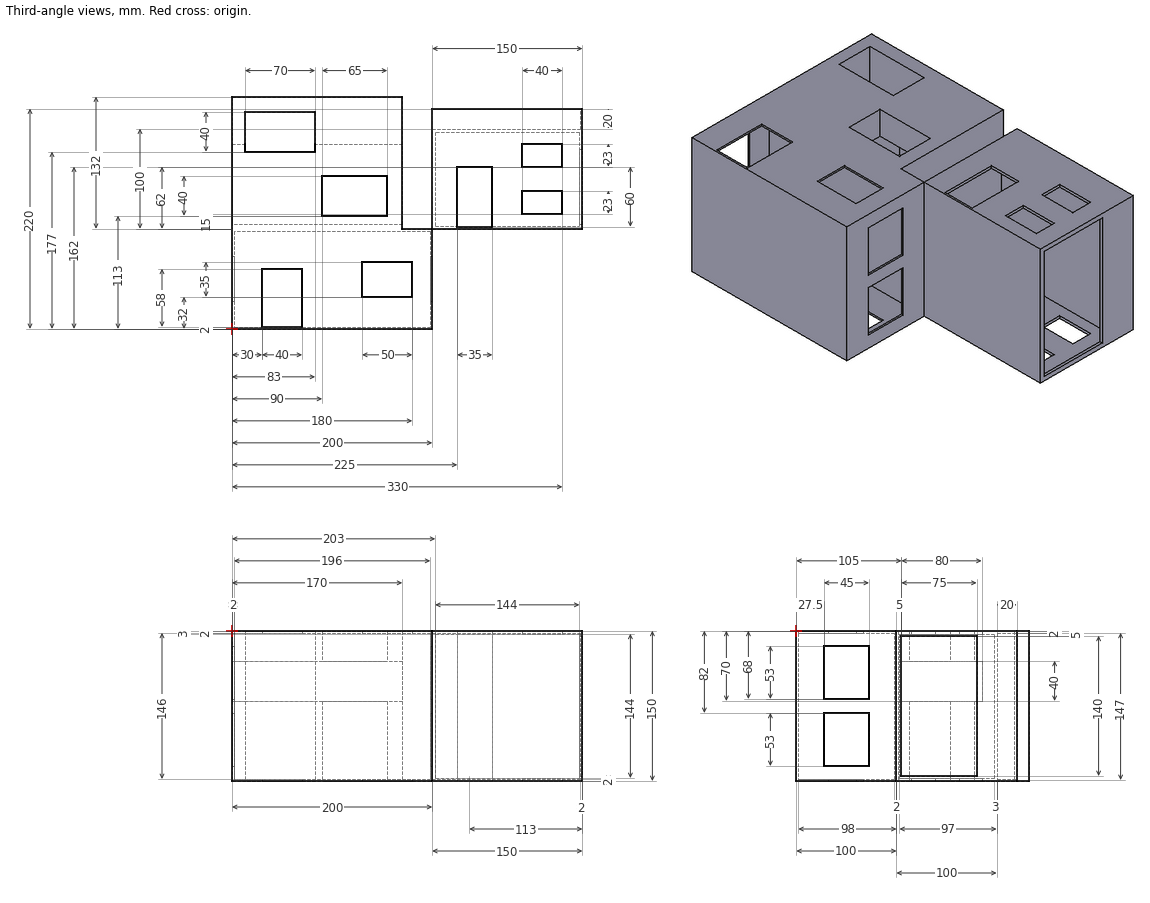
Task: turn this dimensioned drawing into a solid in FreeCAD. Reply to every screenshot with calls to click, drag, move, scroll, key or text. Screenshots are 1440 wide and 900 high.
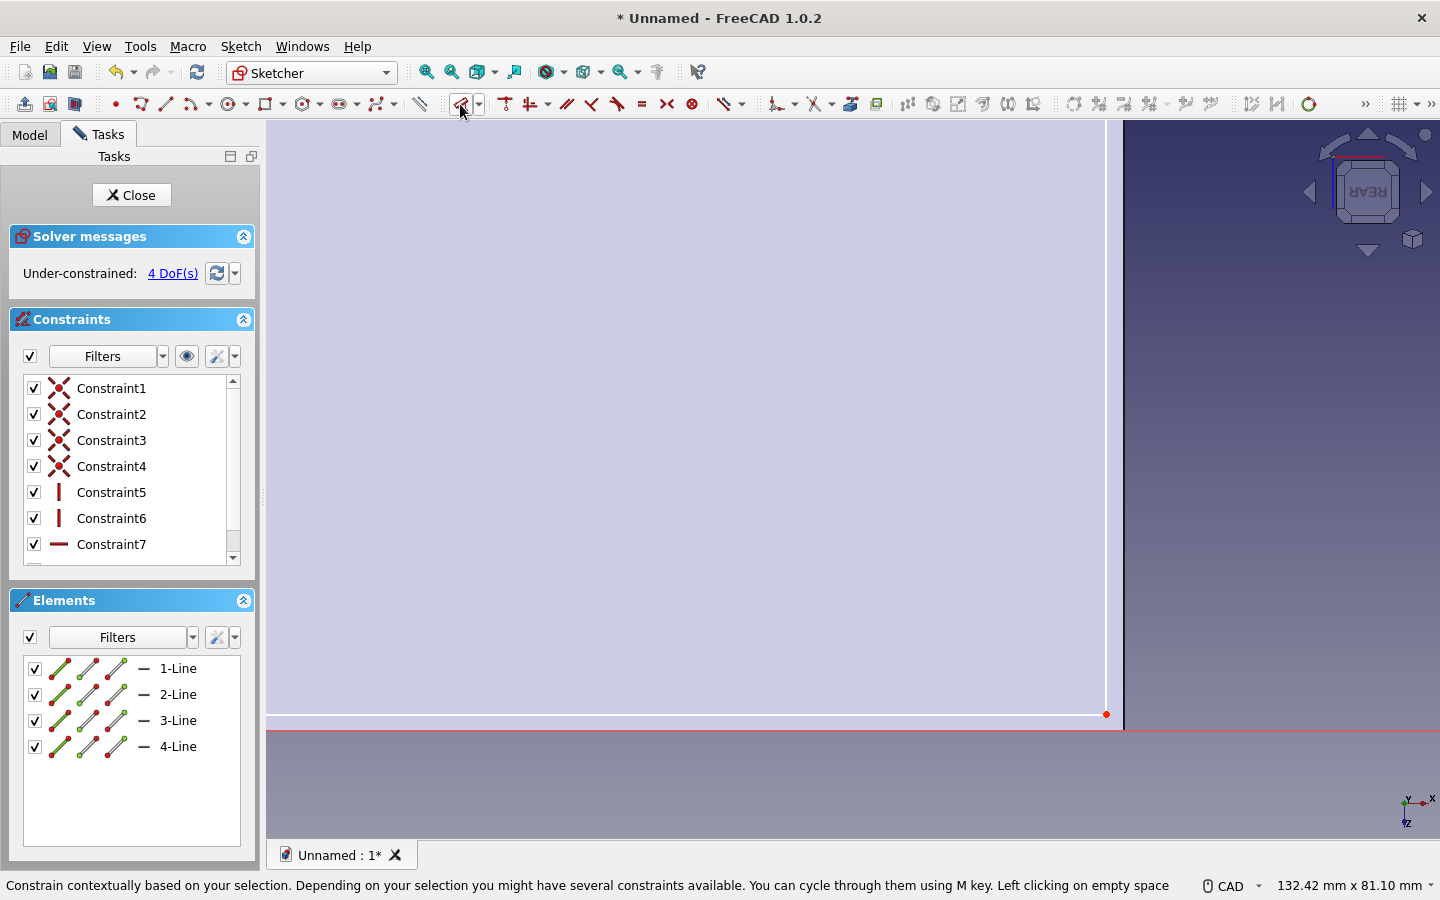
scroll(1108, 715, down, 5)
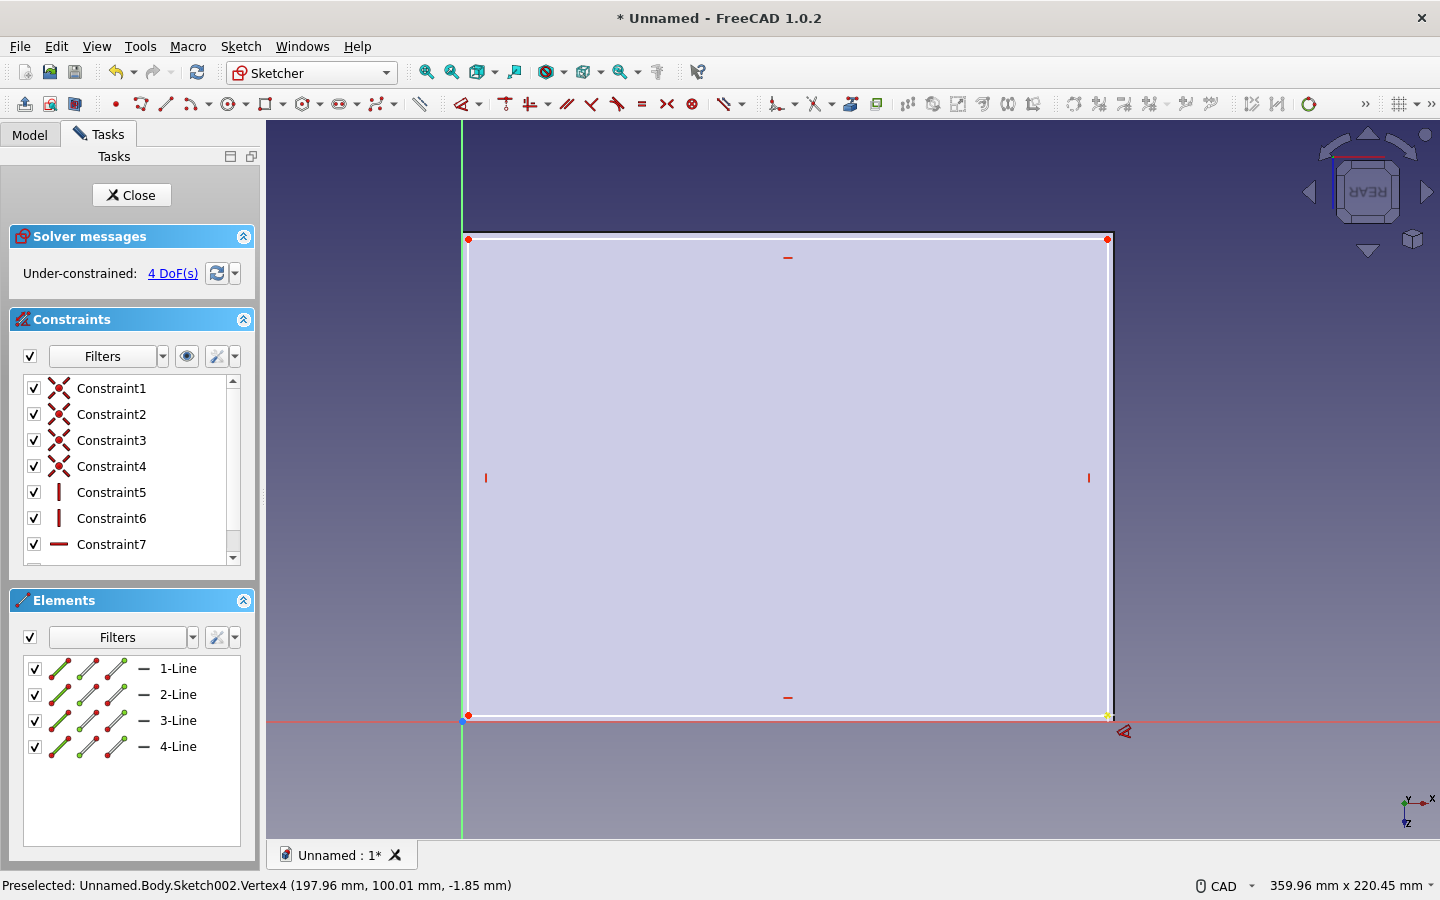
scroll(468, 239, up, 10)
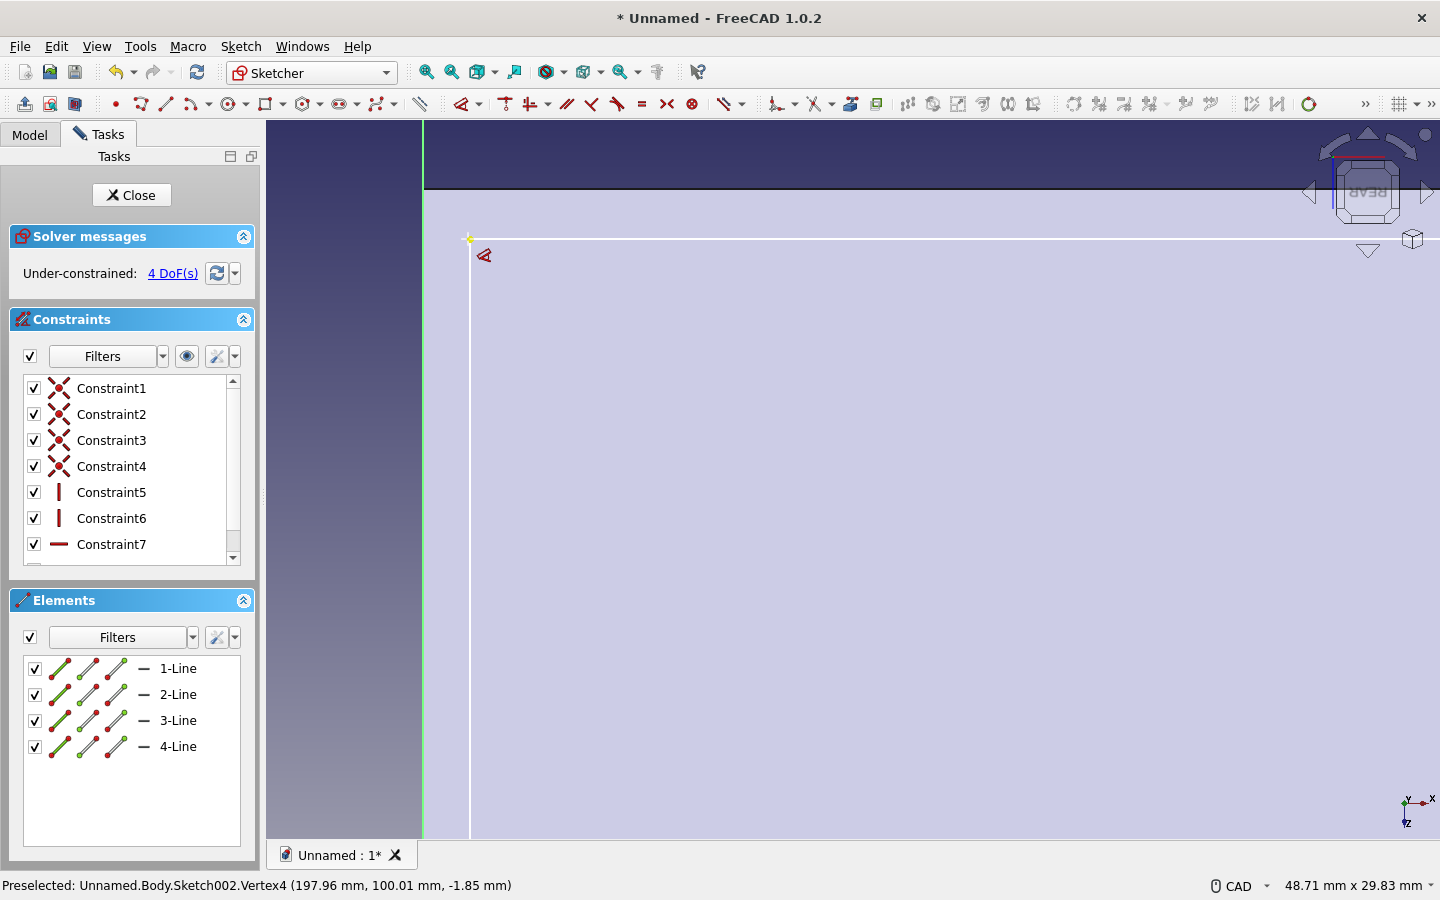
click(470, 239)
click(447, 205)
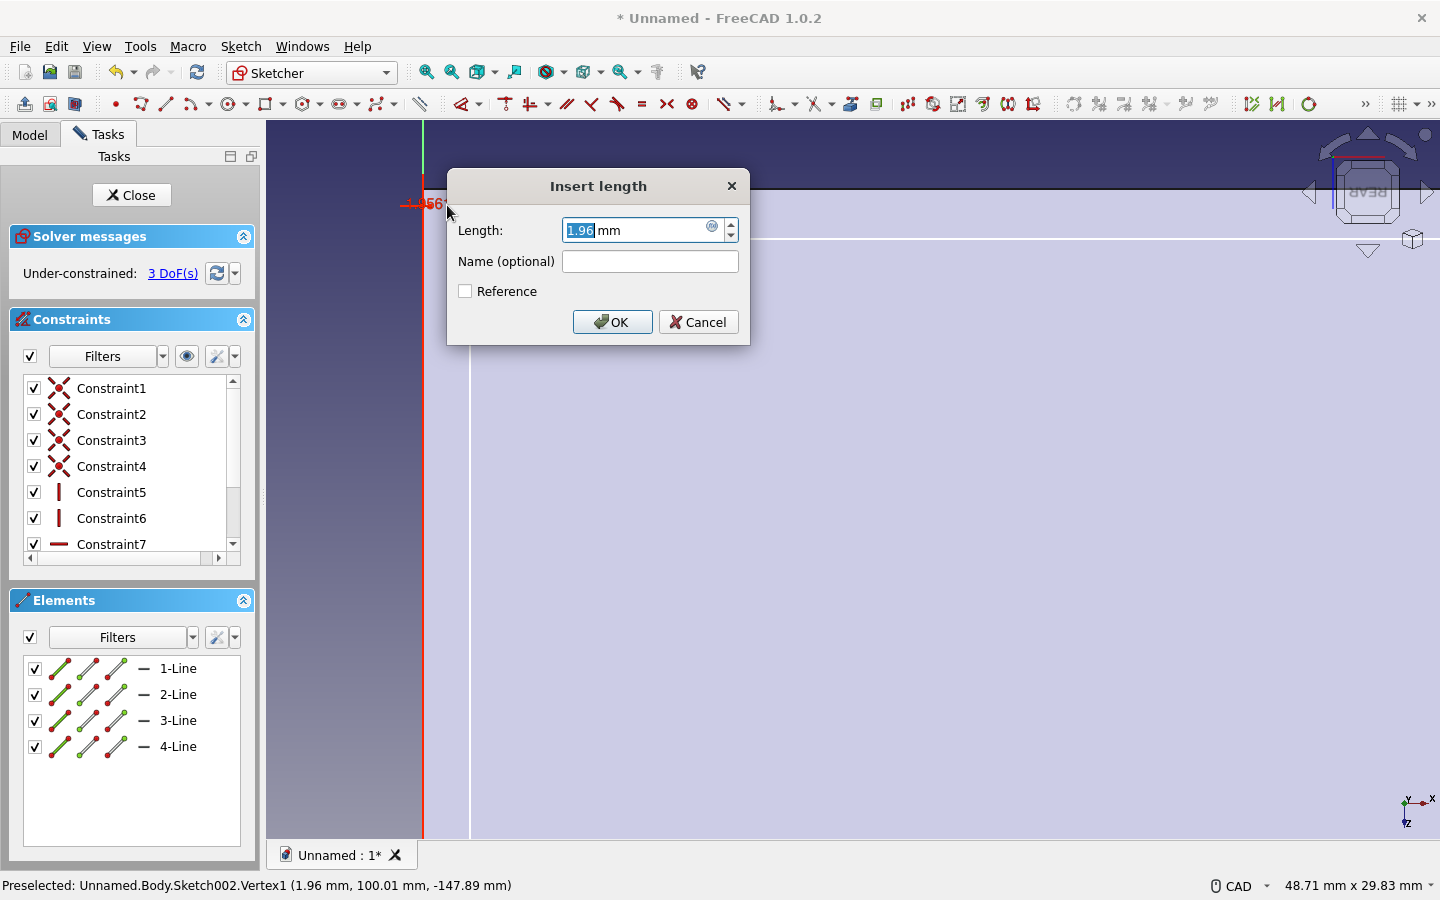
text(2)
key(Return)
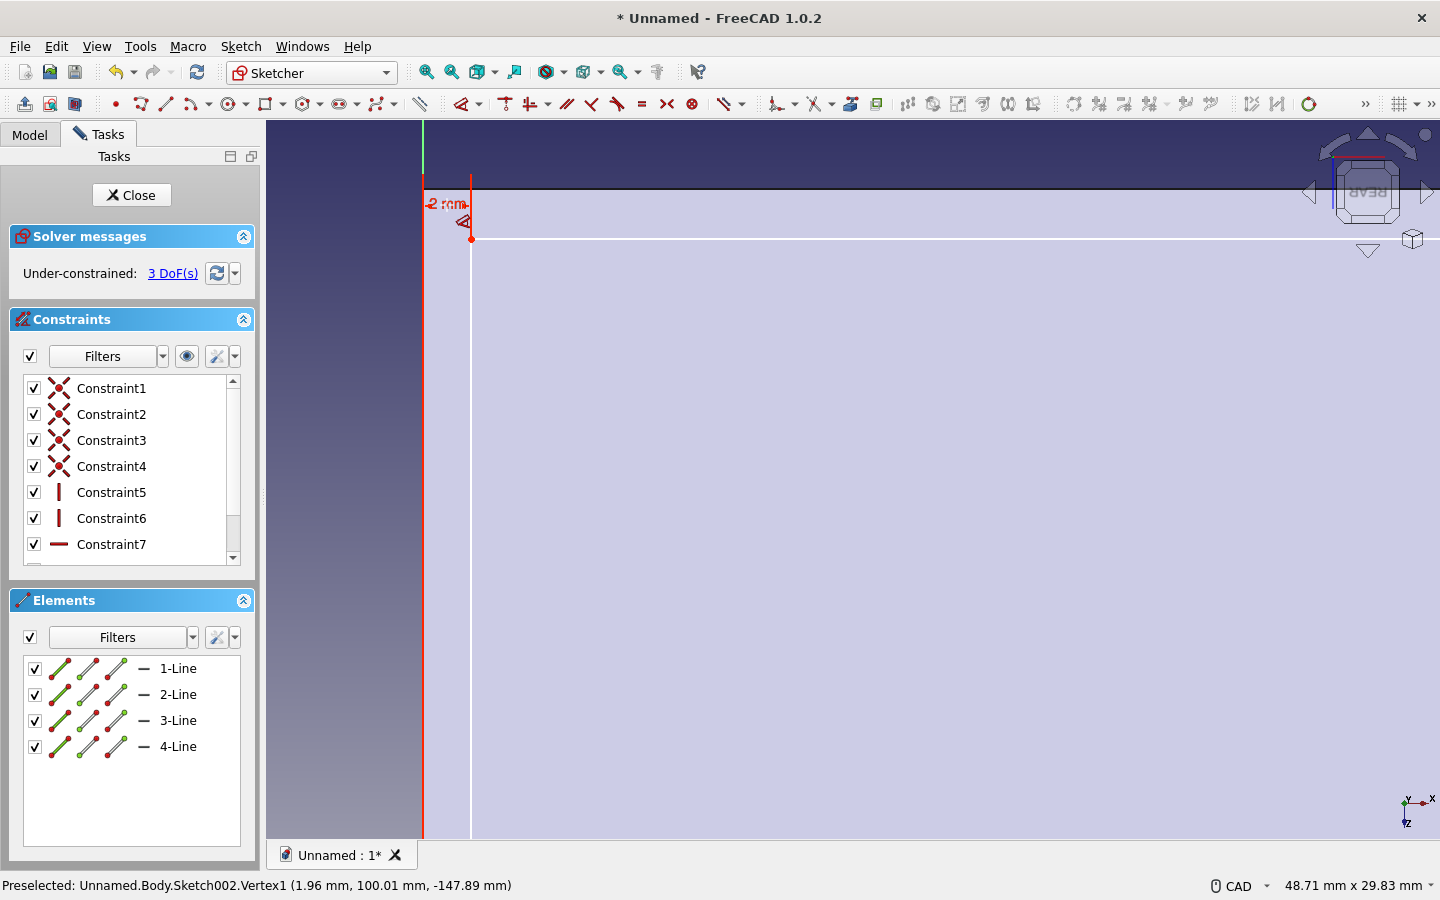
scroll(468, 238, down, 10)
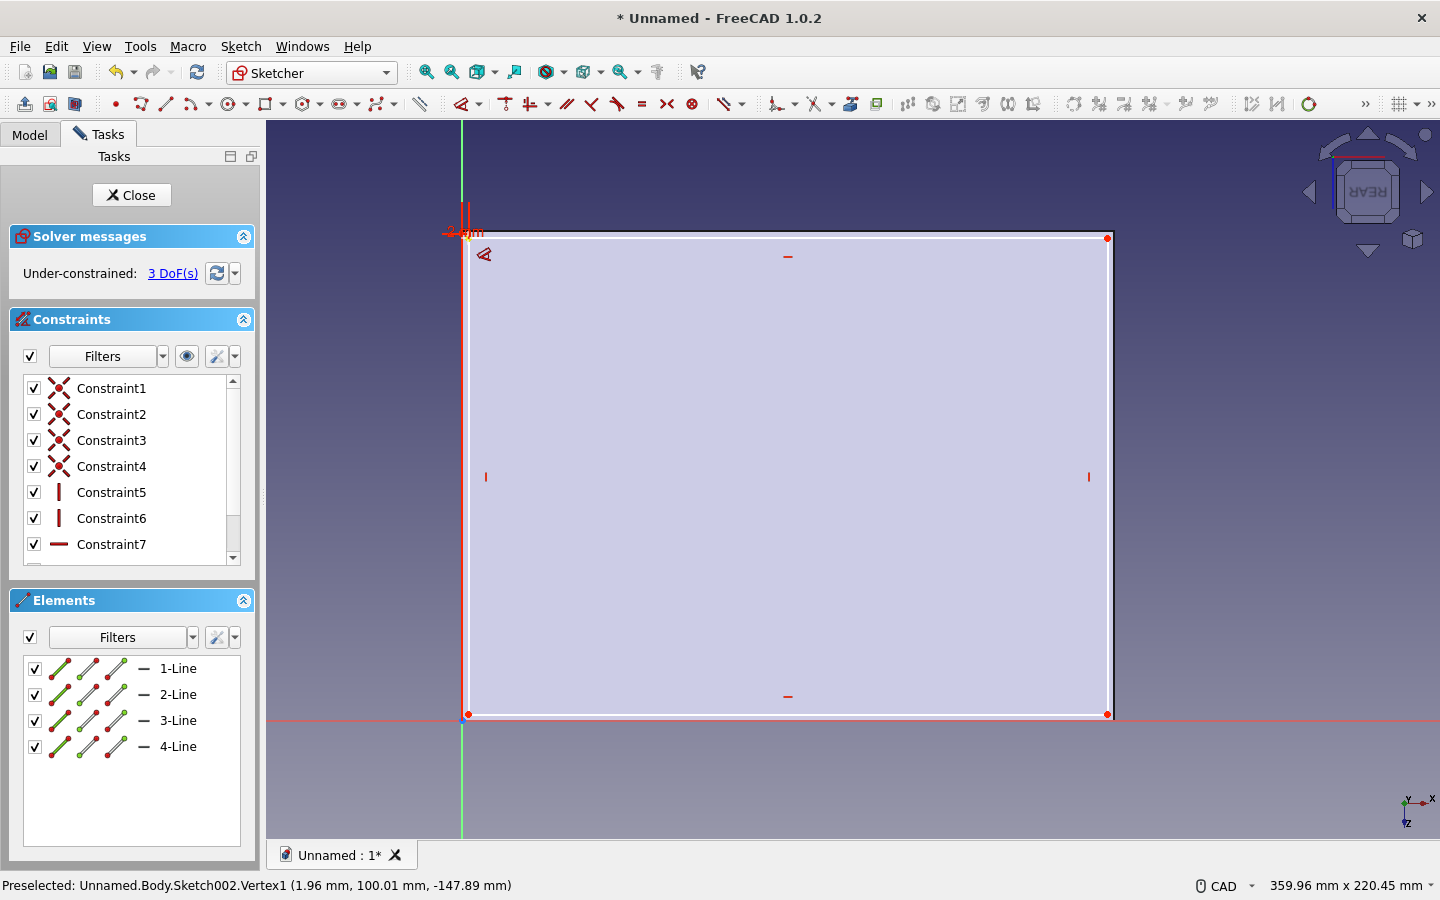
scroll(469, 715, up, 10)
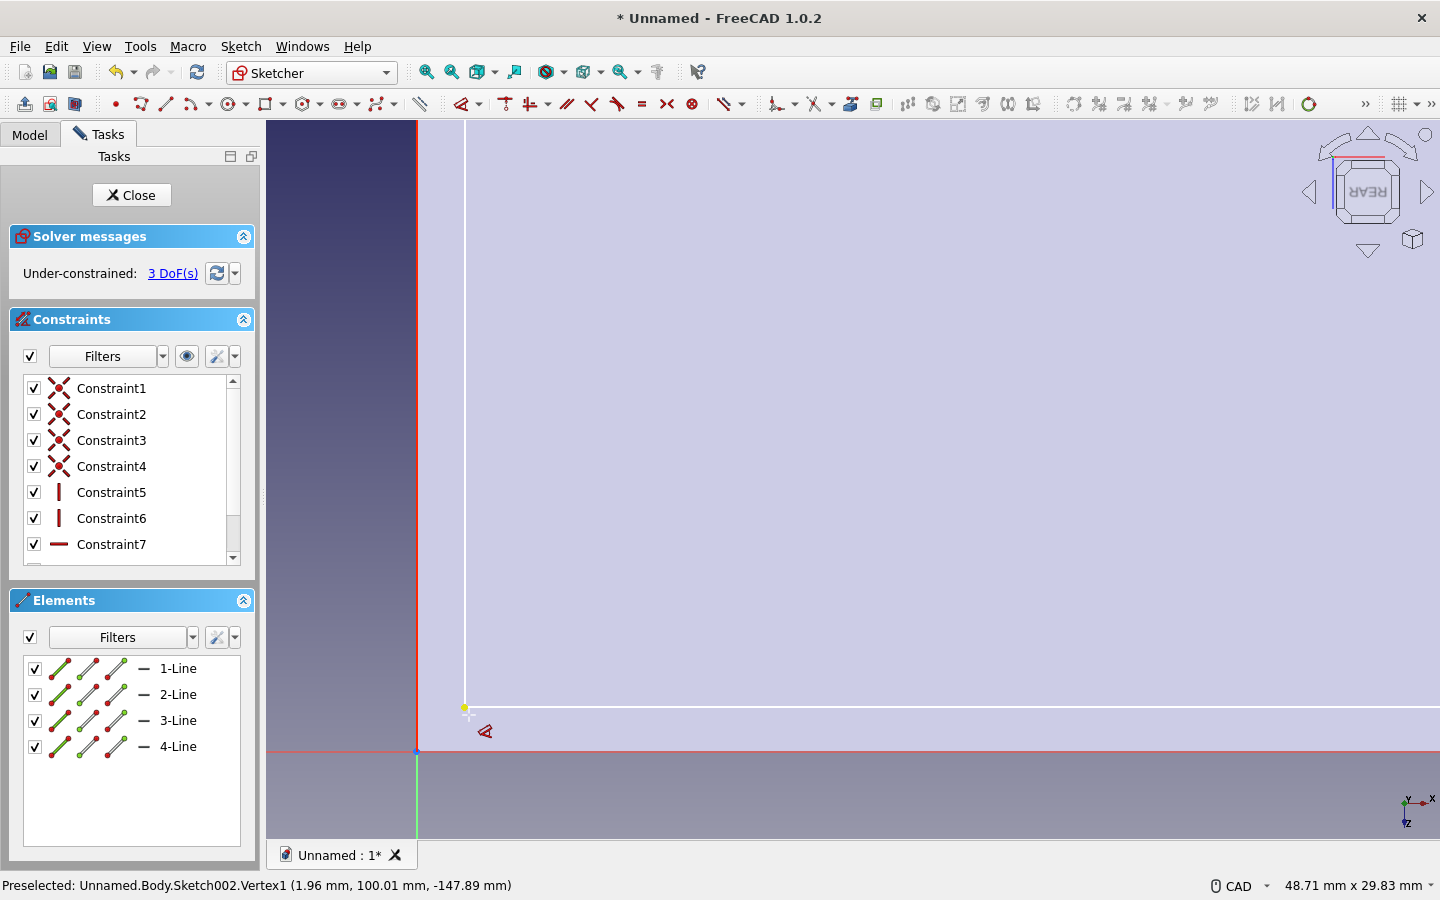
click(465, 707)
click(383, 729)